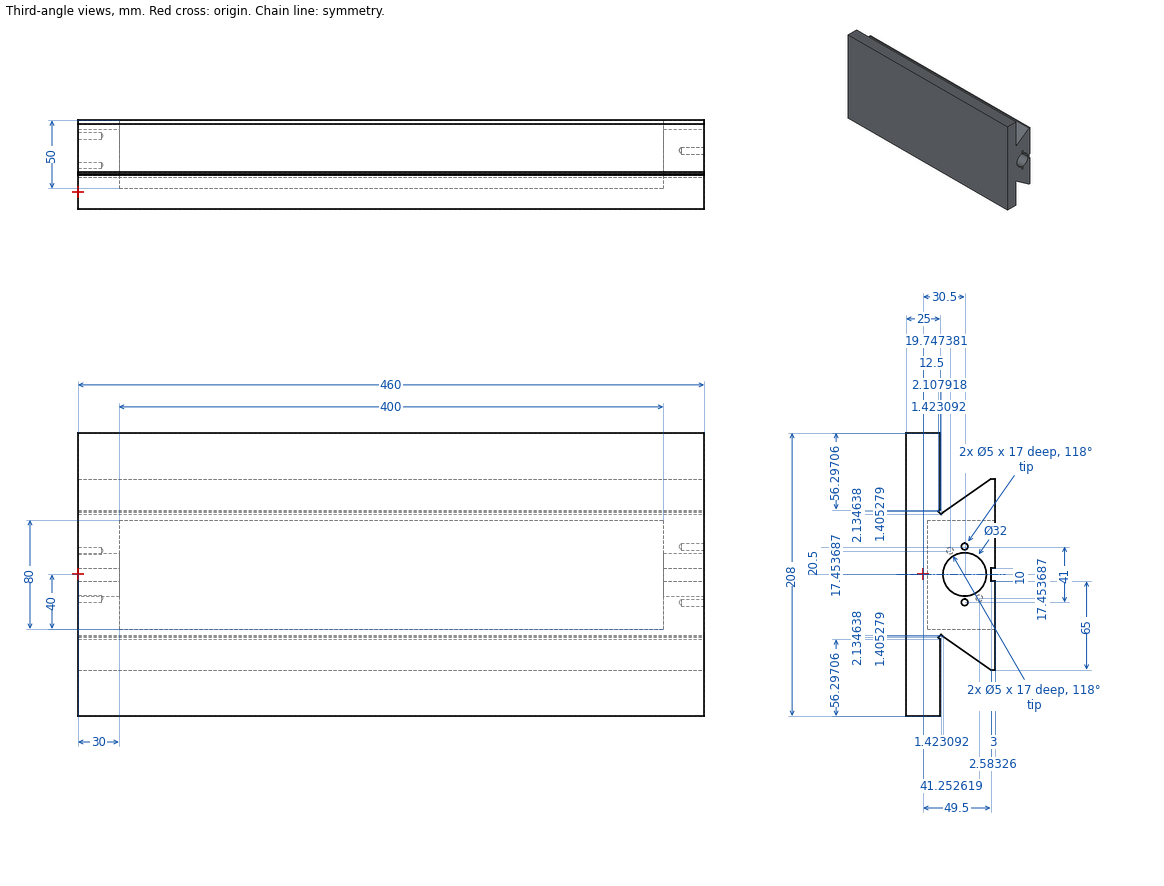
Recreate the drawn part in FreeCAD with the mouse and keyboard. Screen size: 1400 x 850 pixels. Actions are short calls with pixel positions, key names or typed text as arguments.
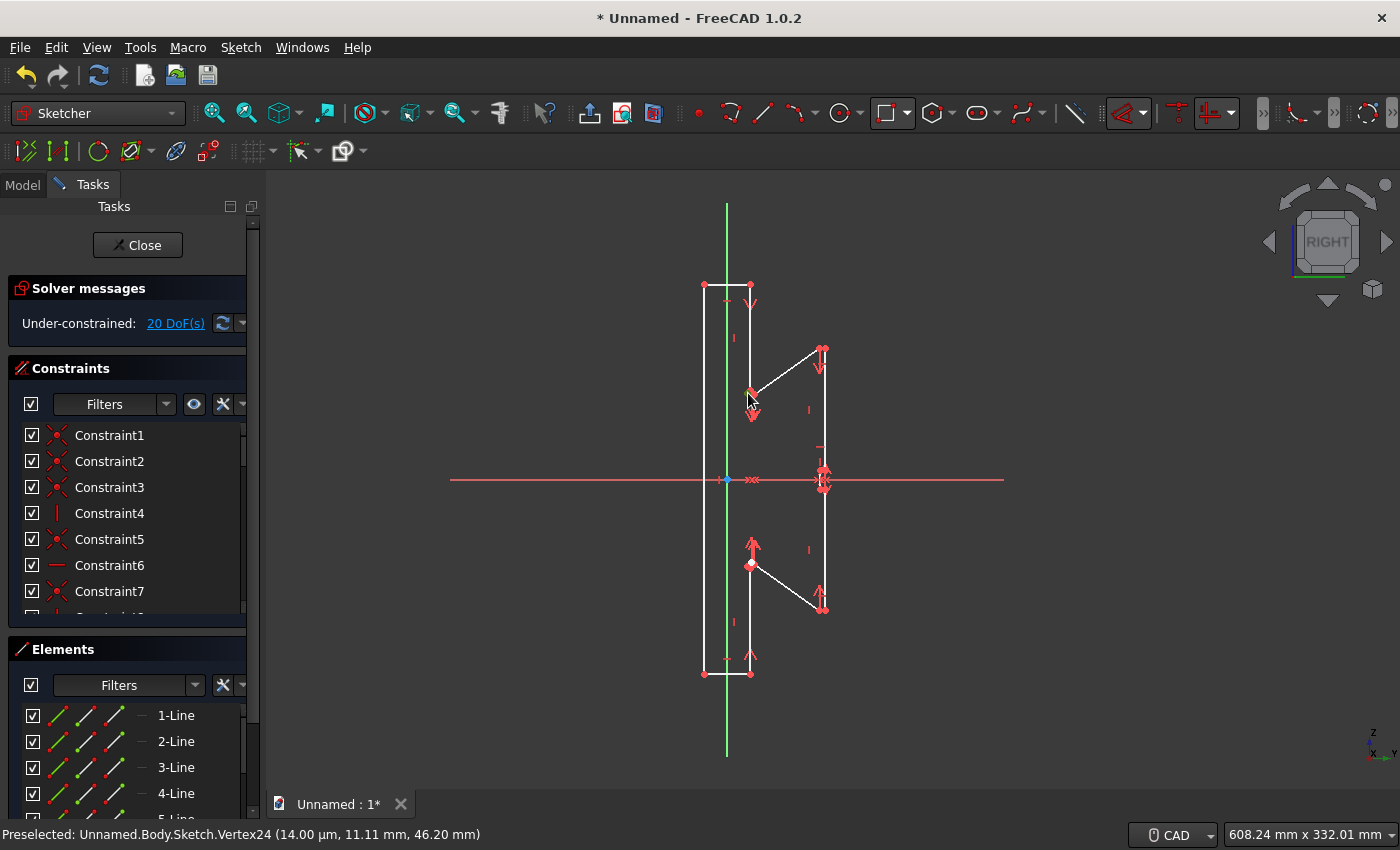
scroll(748, 566, up, 6)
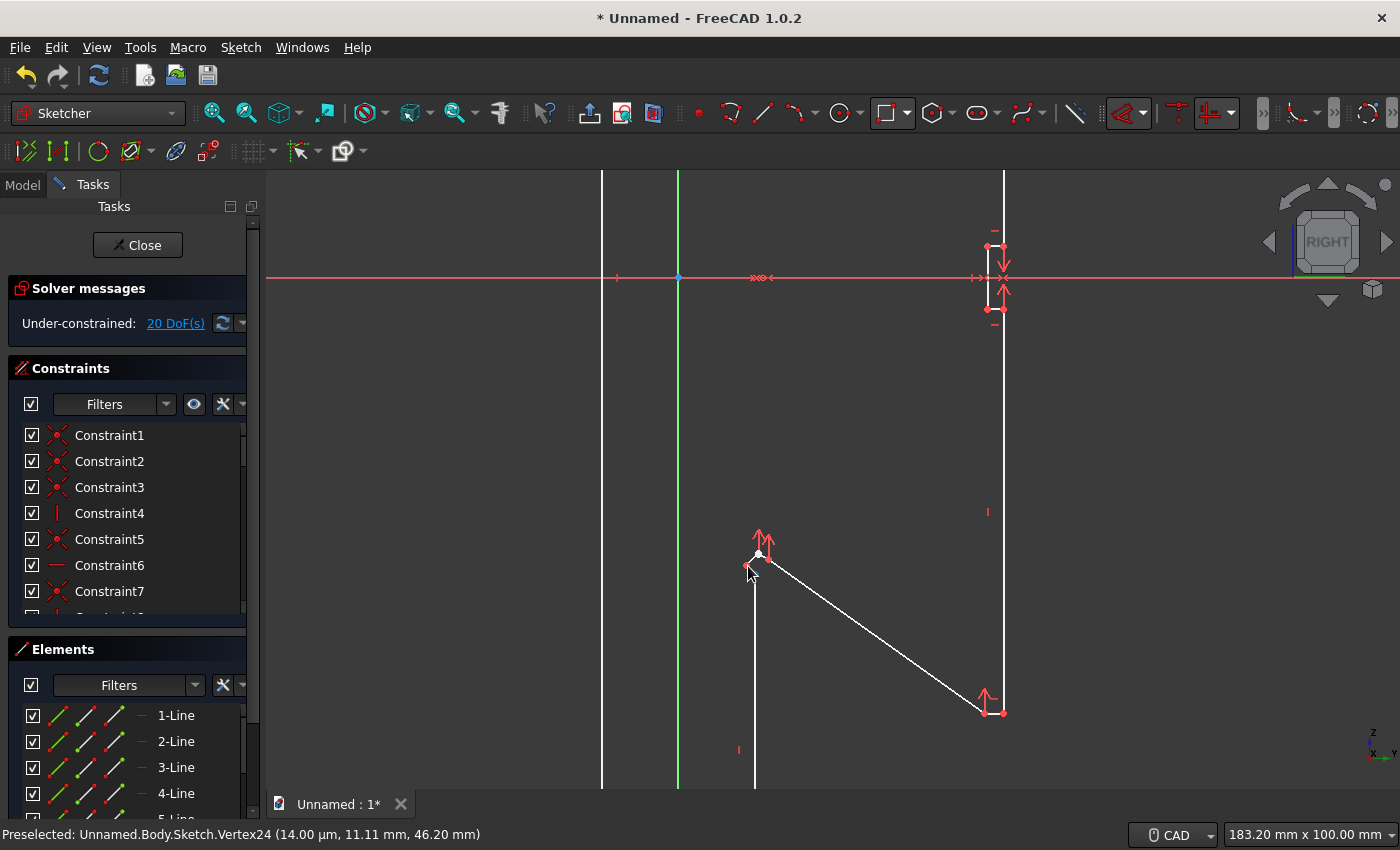
click(747, 565)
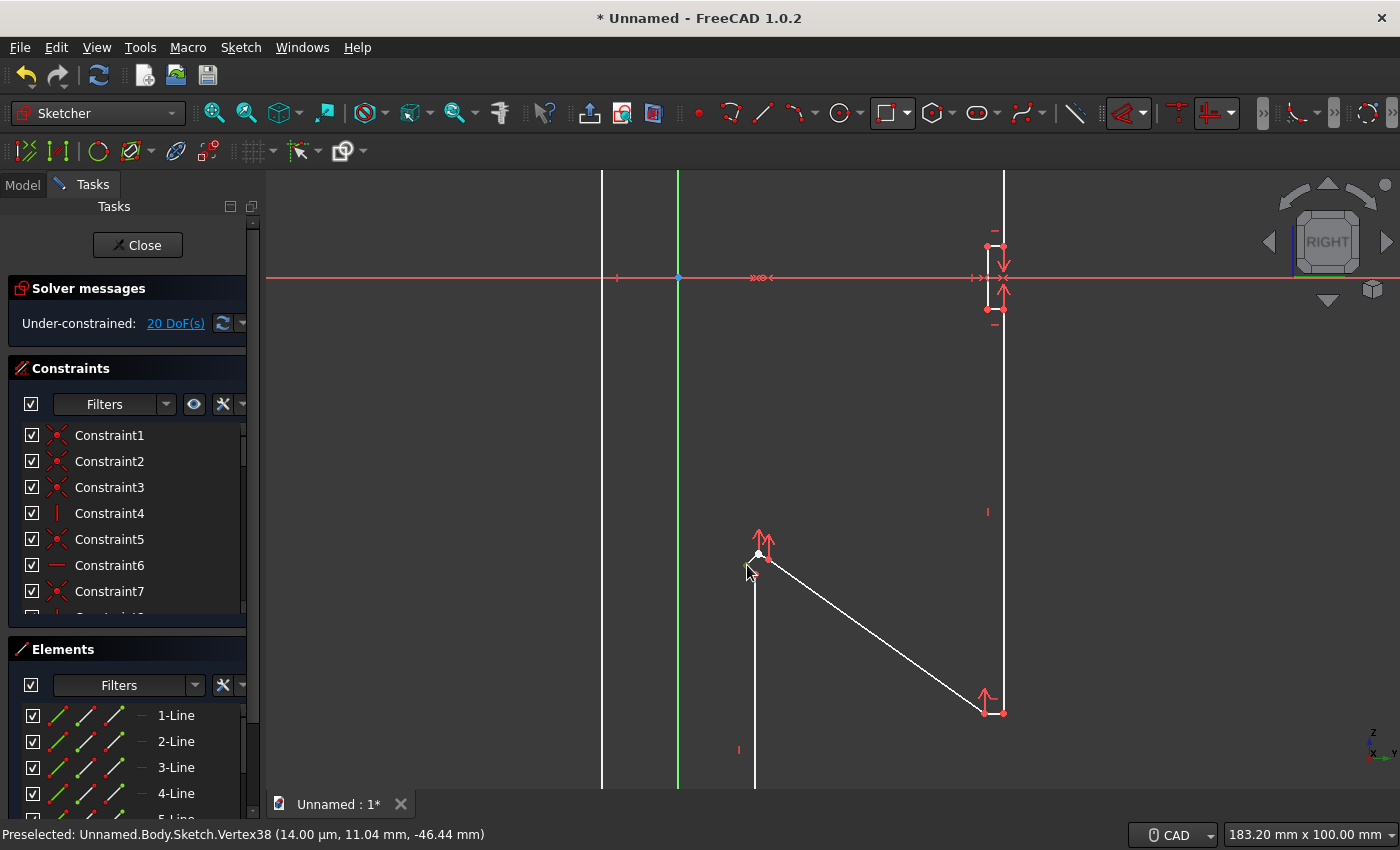
click(361, 278)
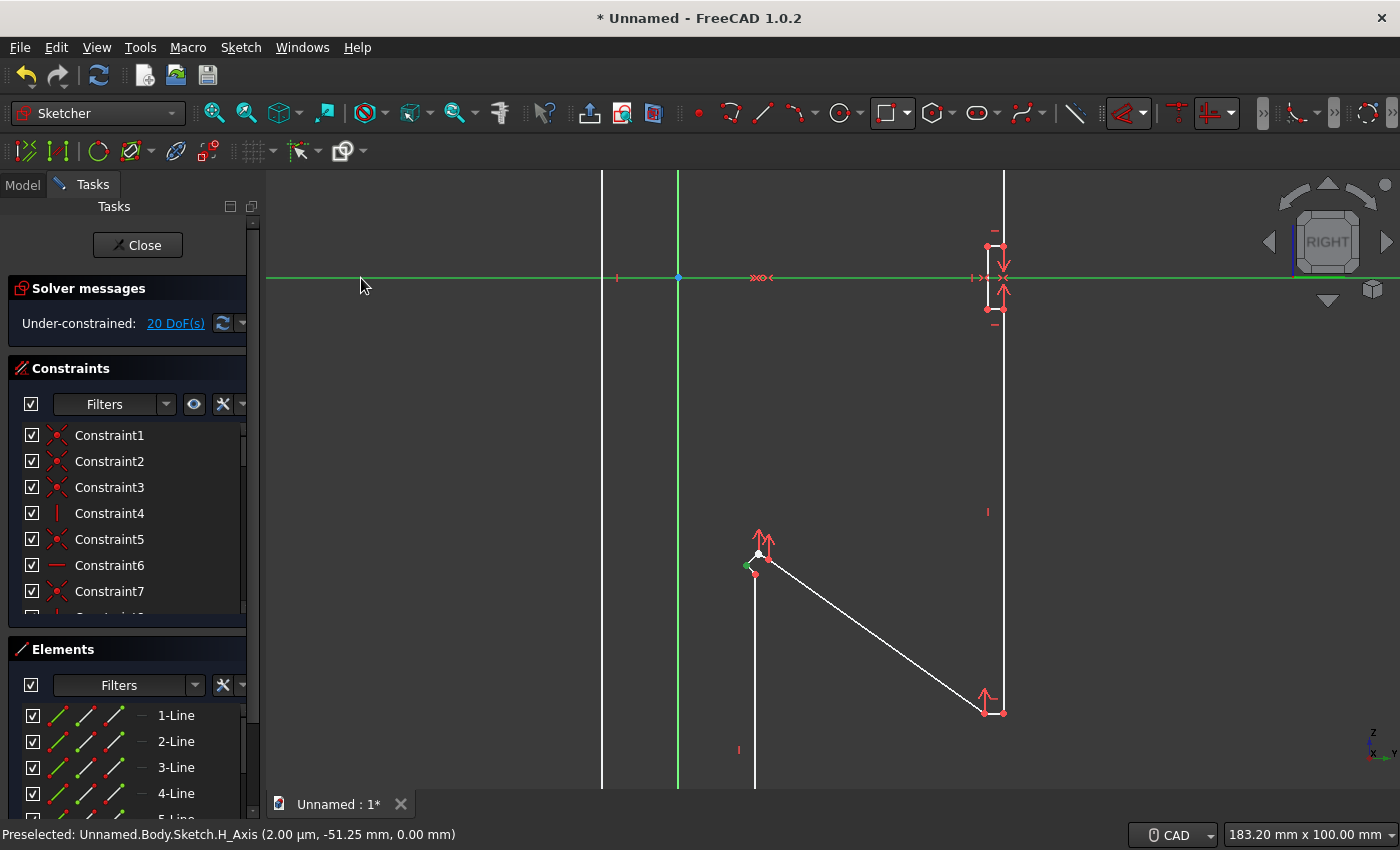
key(s)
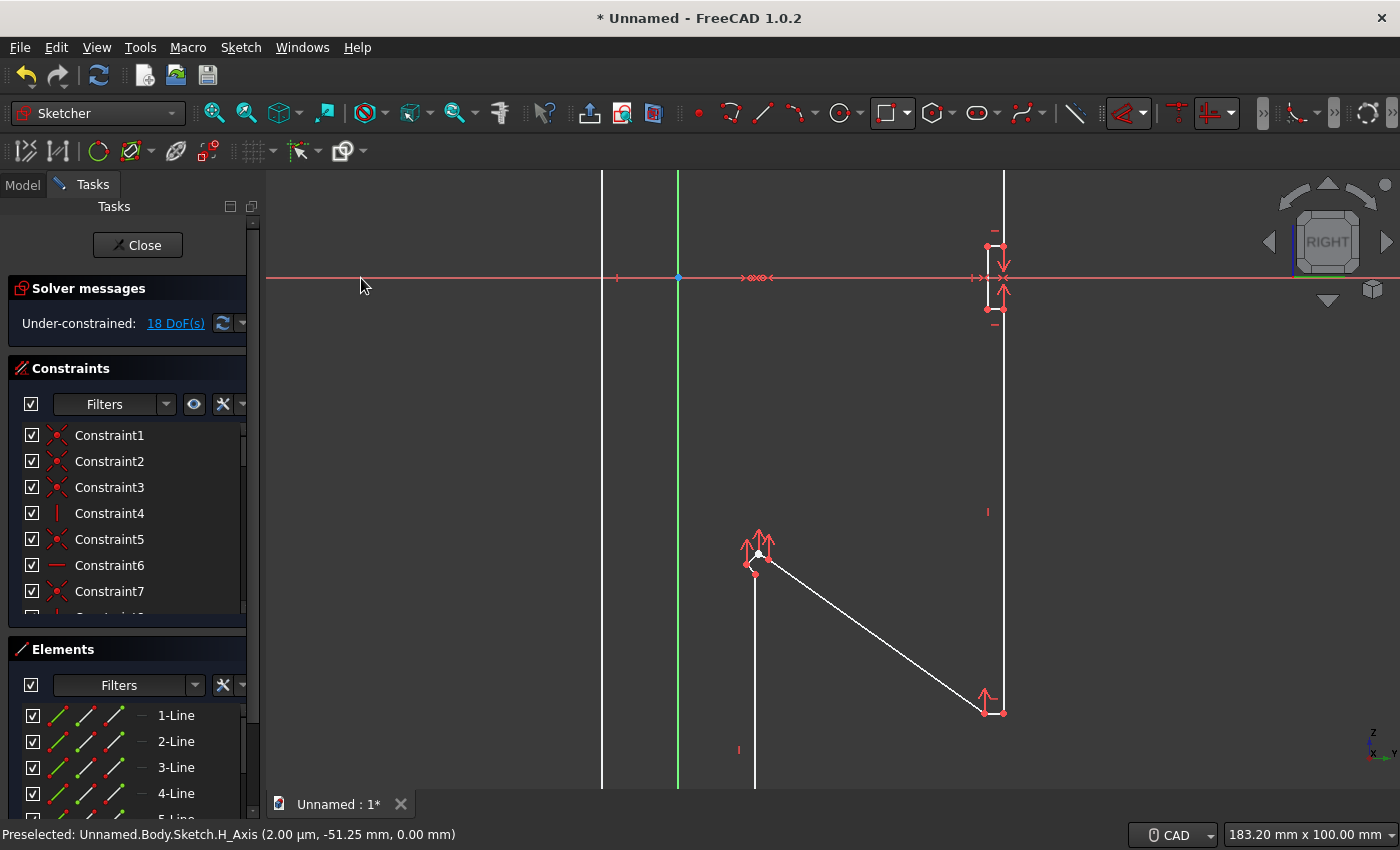
click(1122, 114)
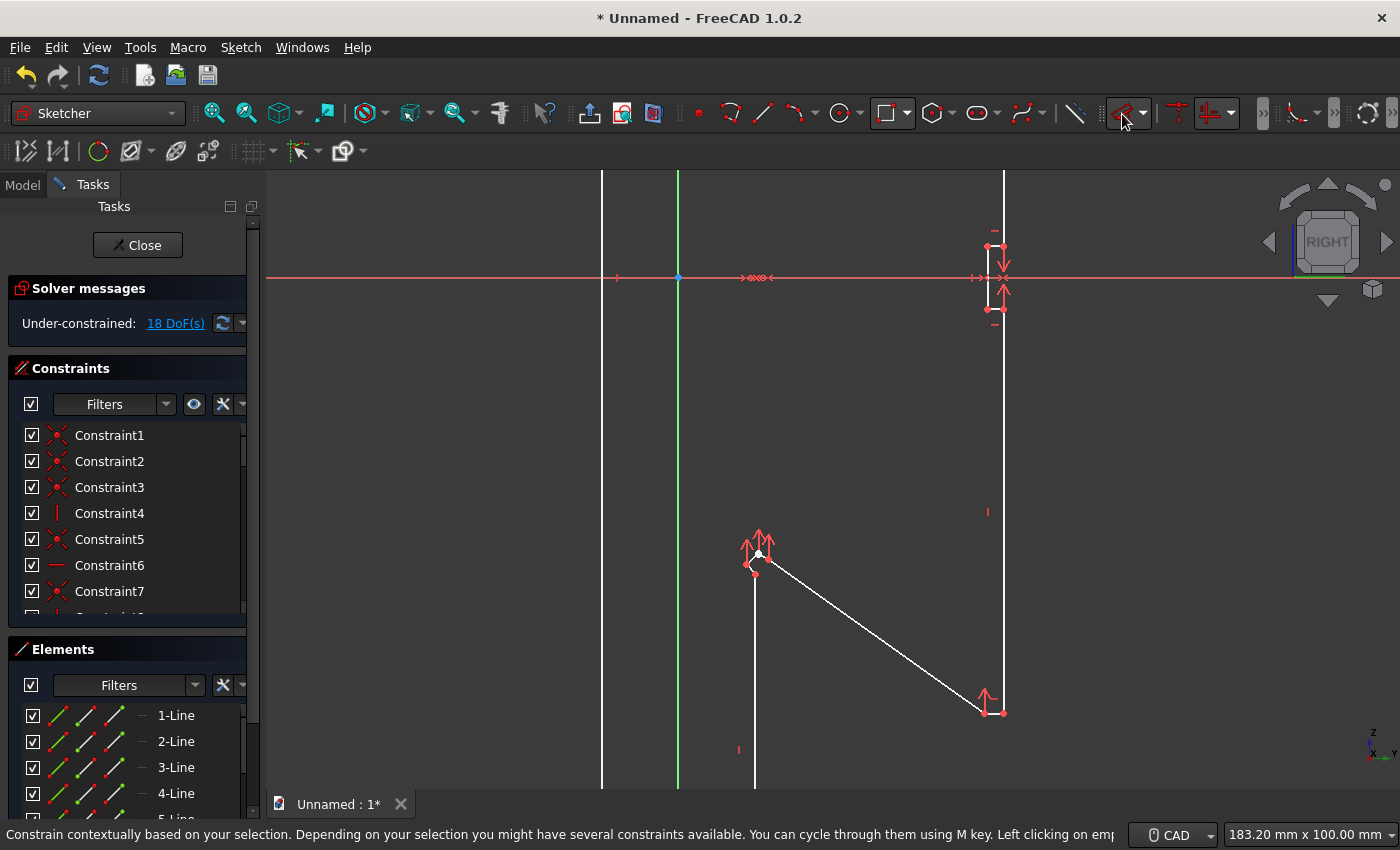
scroll(994, 714, up, 4)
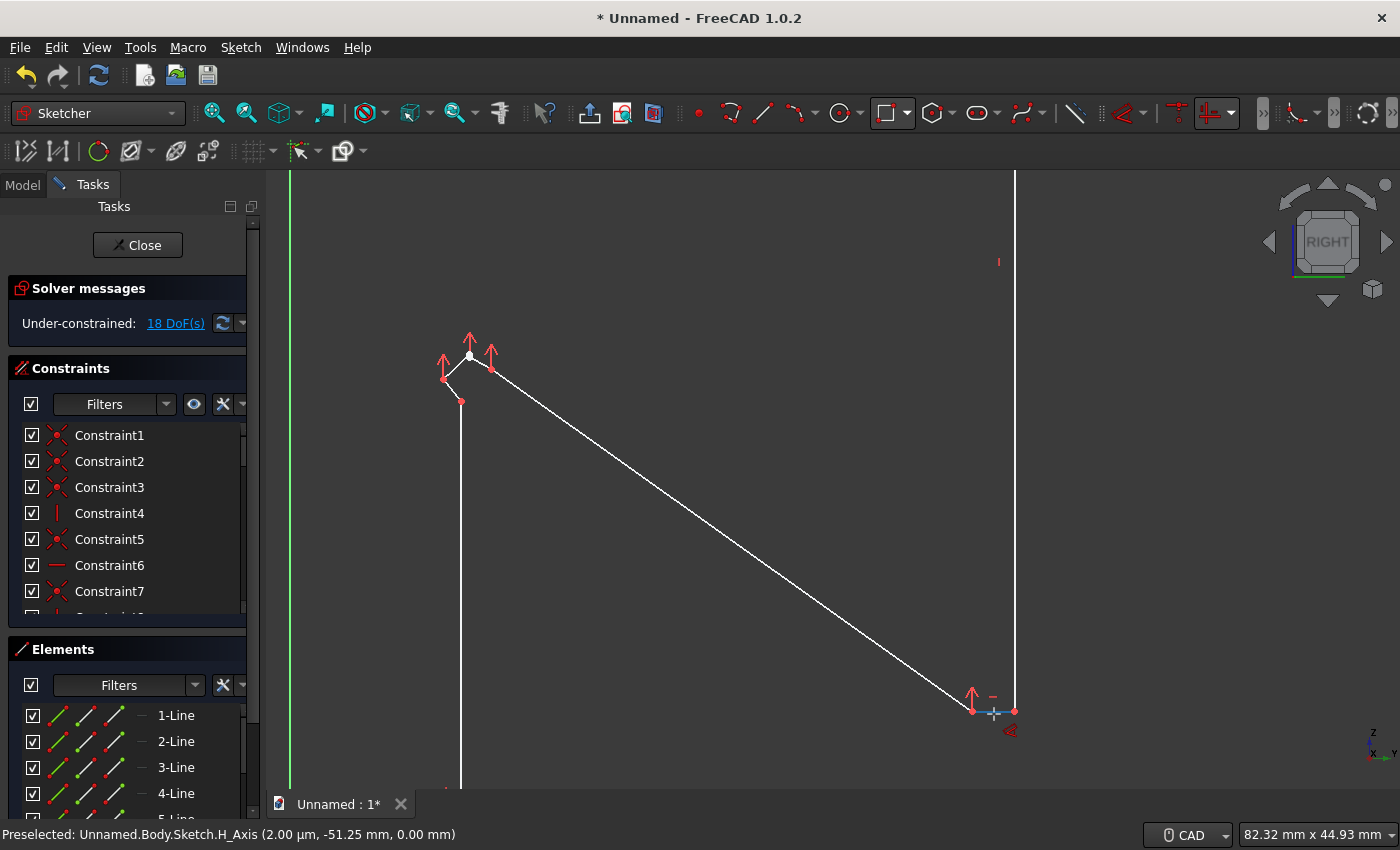
click(993, 712)
click(993, 746)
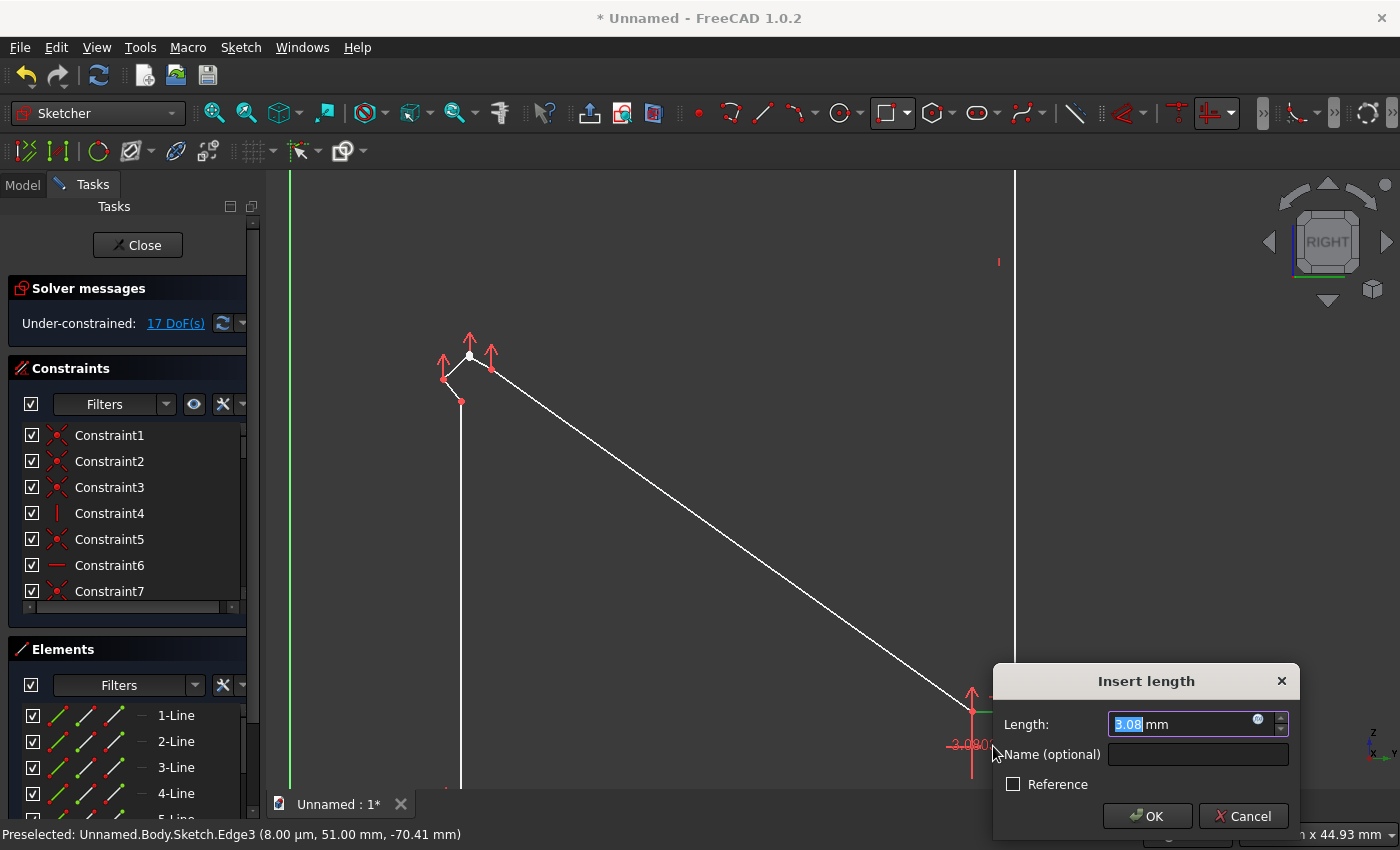
text(3)
key(Return)